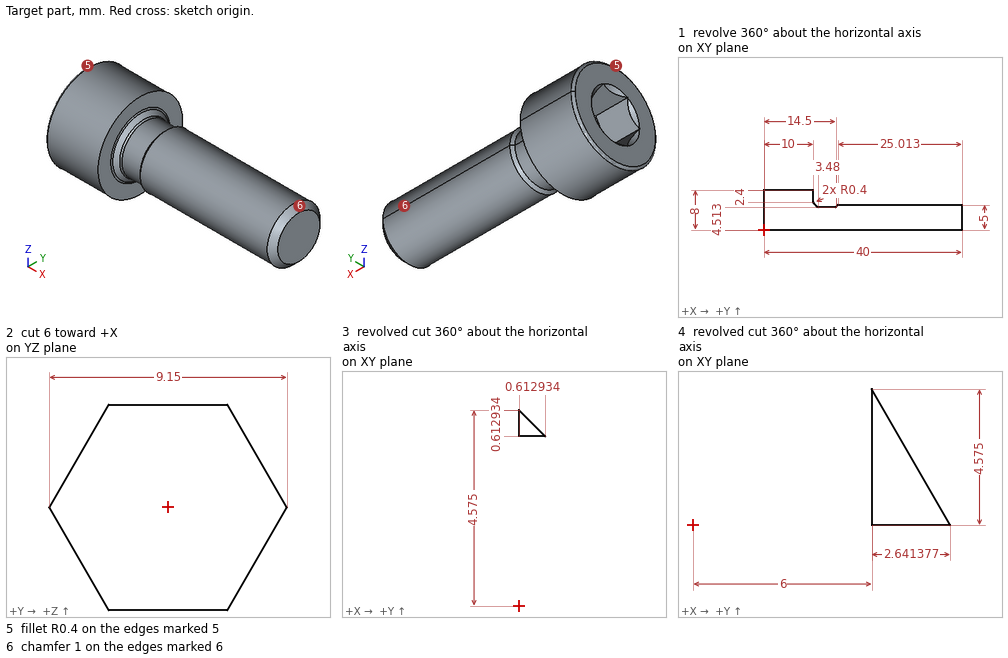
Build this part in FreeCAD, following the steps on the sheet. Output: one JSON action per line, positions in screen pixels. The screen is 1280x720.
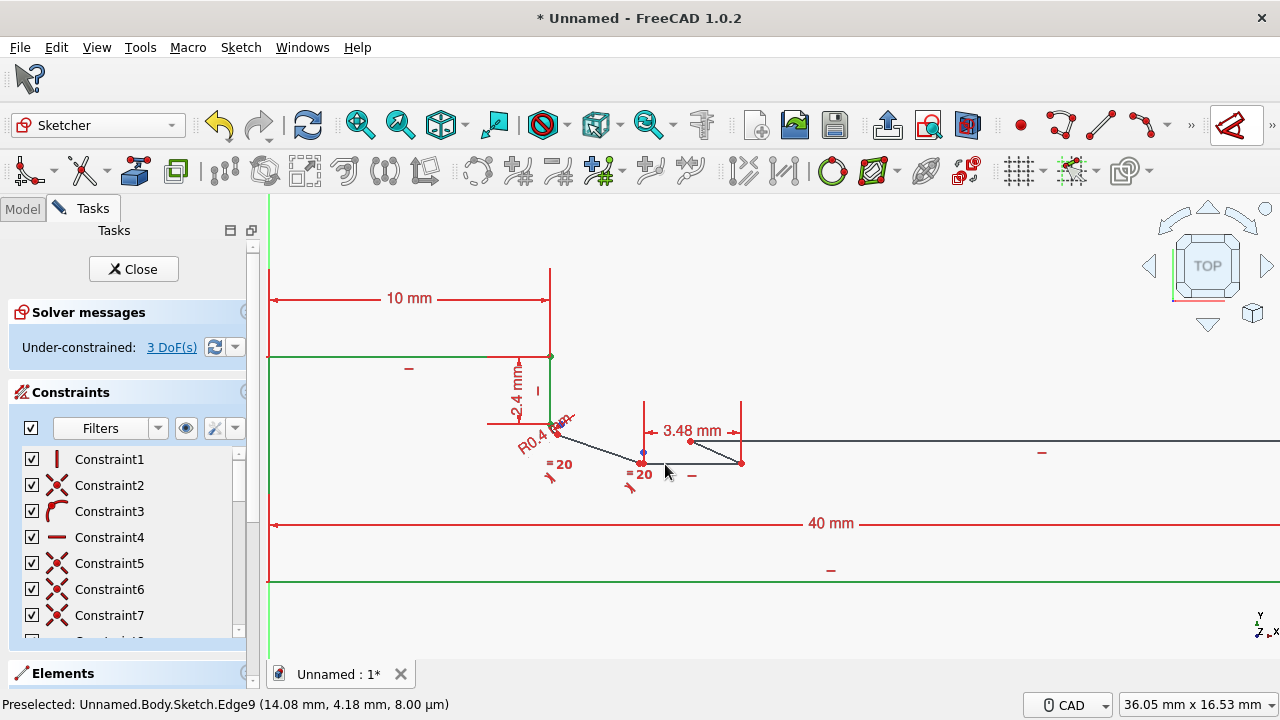
{"action": "left_click", "coordinate": [741, 464]}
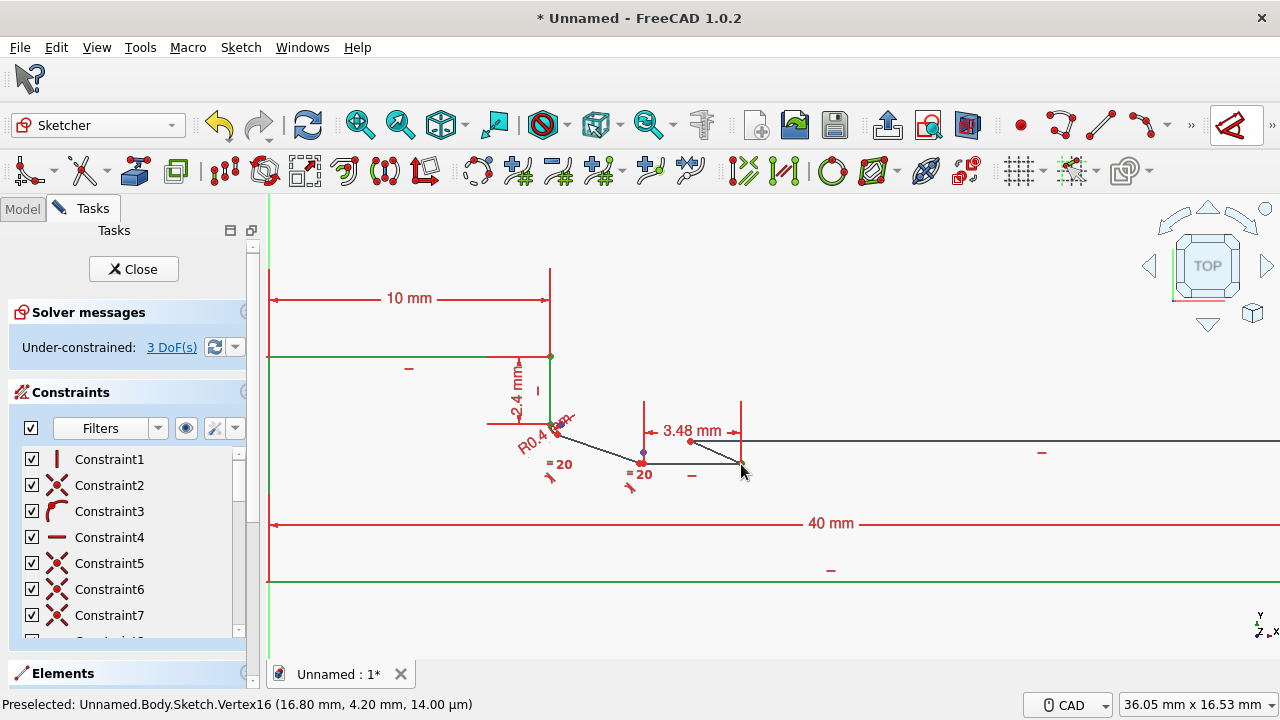
{"action": "key", "text": "l"}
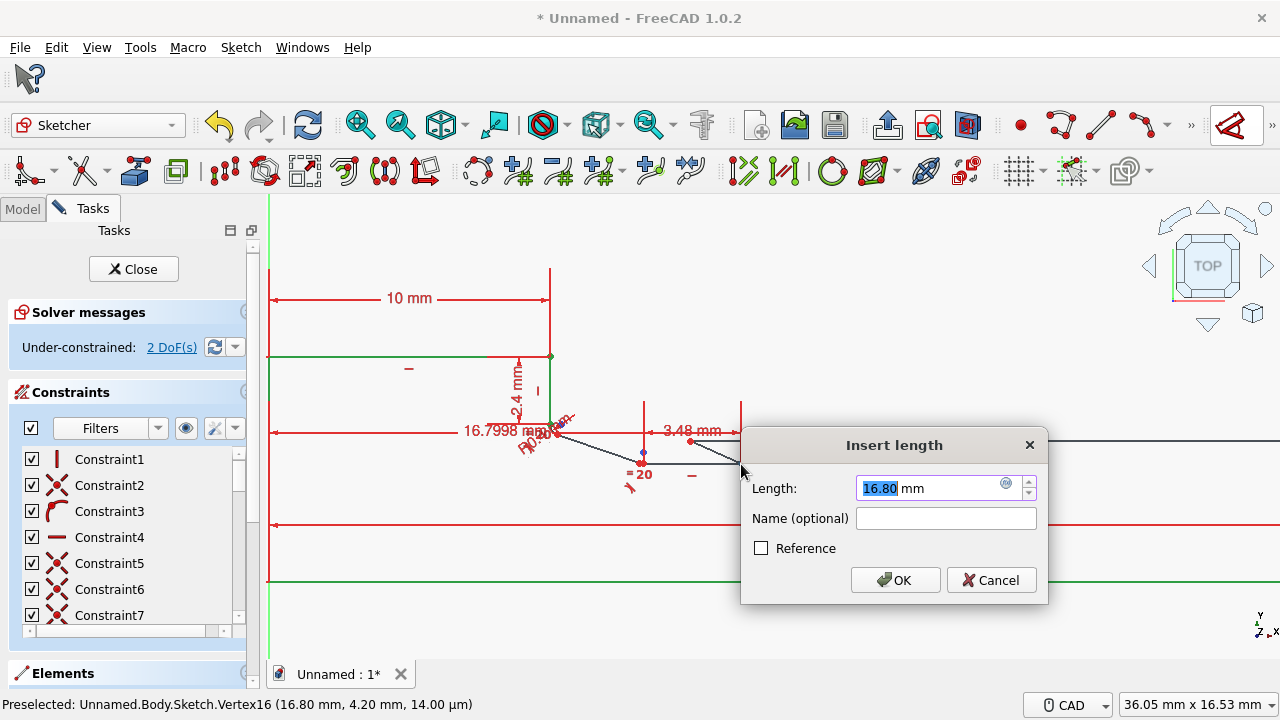
{"action": "type", "text": "14.5"}
{"action": "key", "text": "Return"}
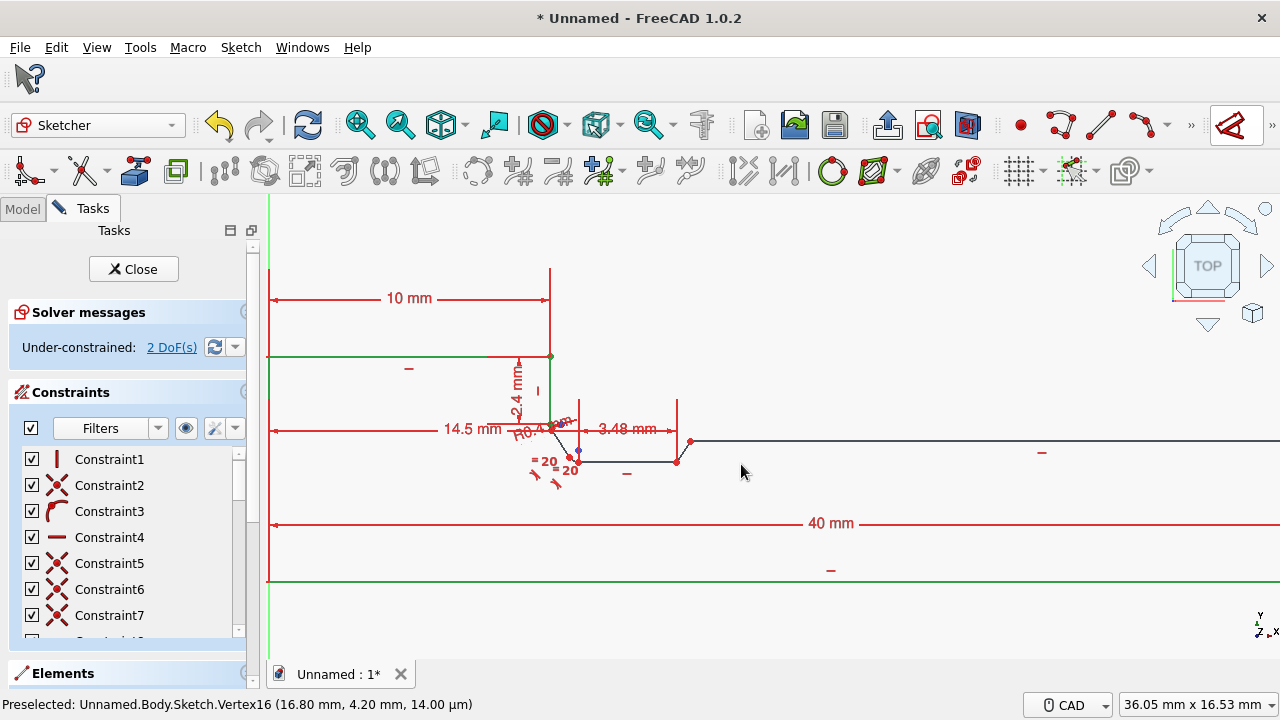
{"action": "left_click", "coordinate": [902, 441]}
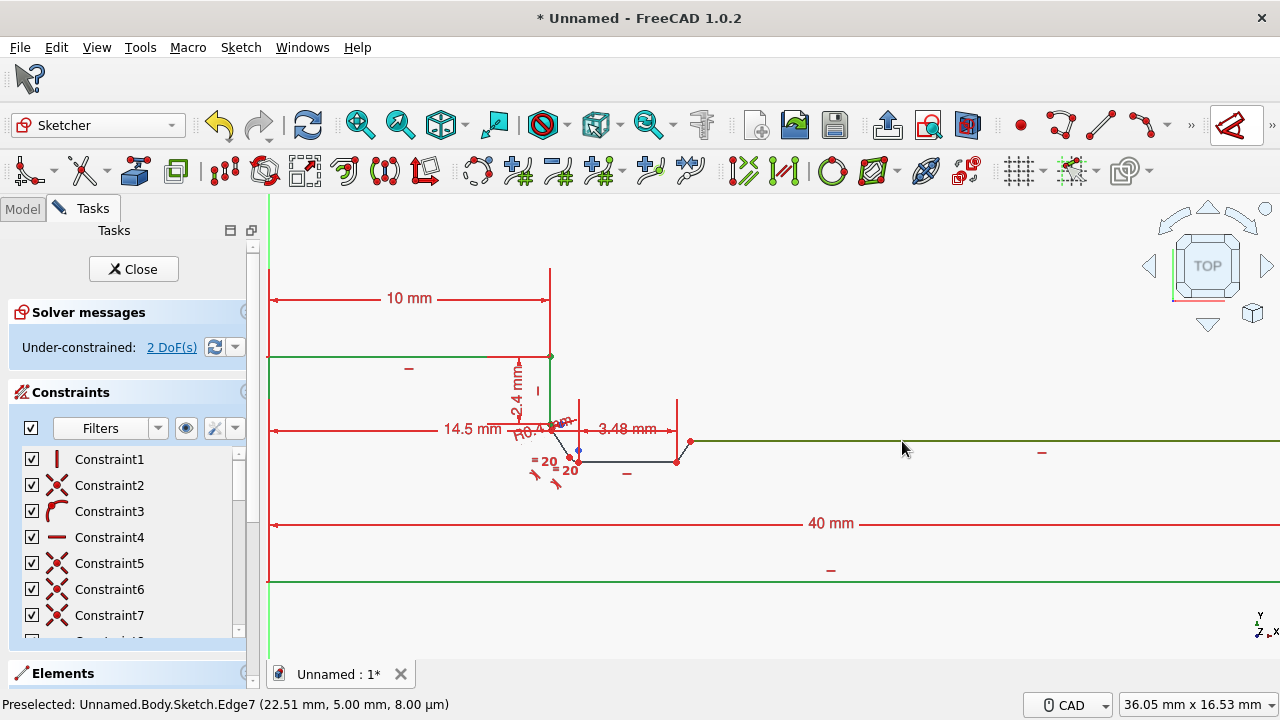
{"action": "left_click", "coordinate": [1258, 126]}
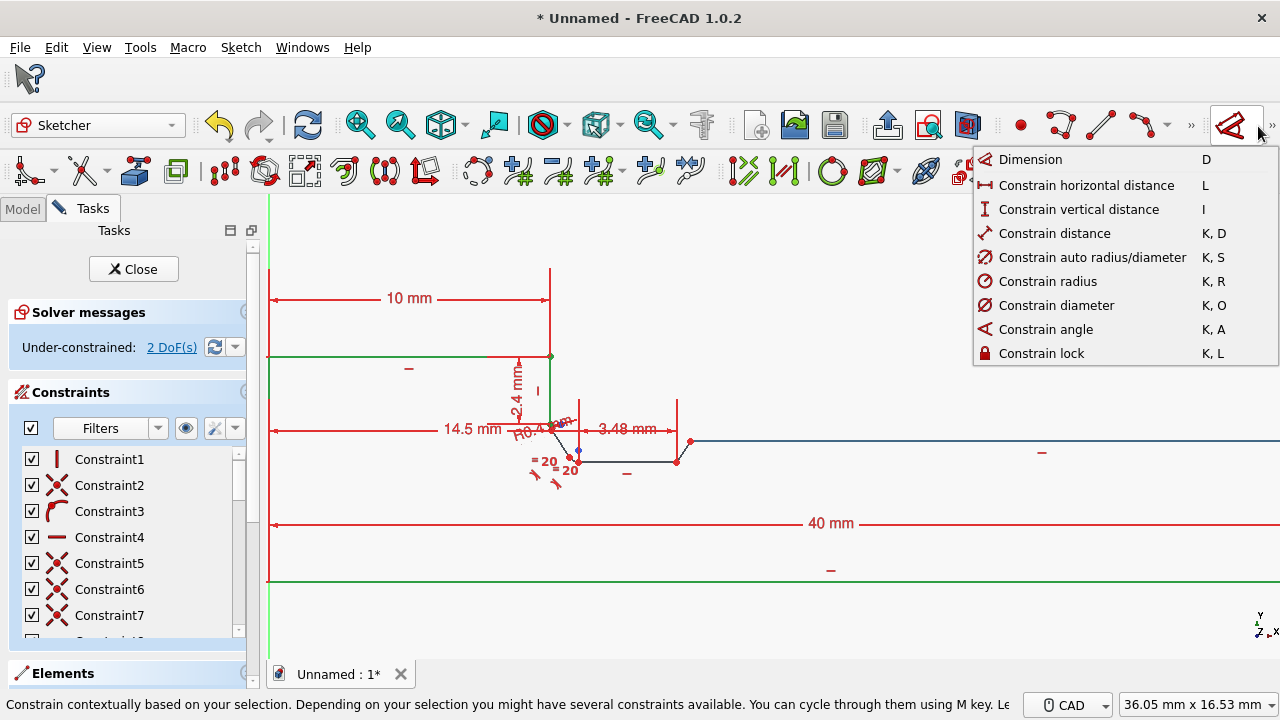
{"action": "left_click", "coordinate": [1126, 185]}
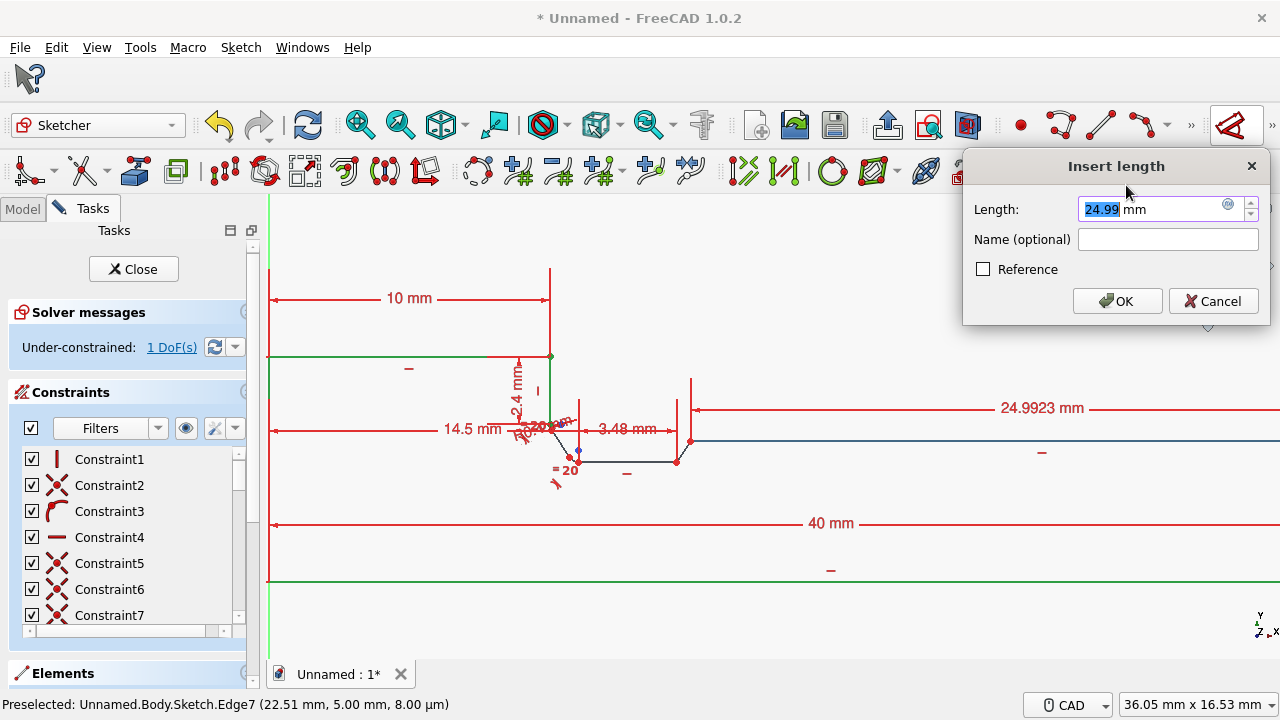
{"action": "type", "text": "25.013"}
{"action": "key", "text": "Return"}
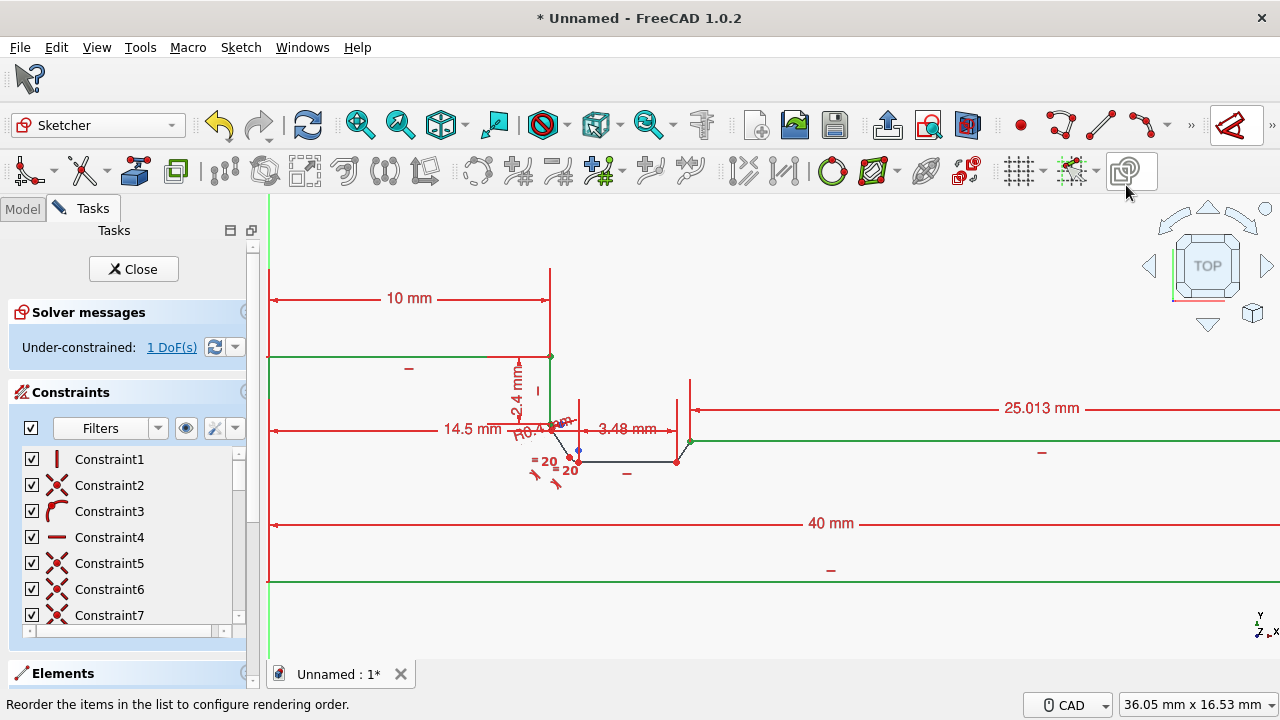
{"action": "left_click", "coordinate": [677, 462]}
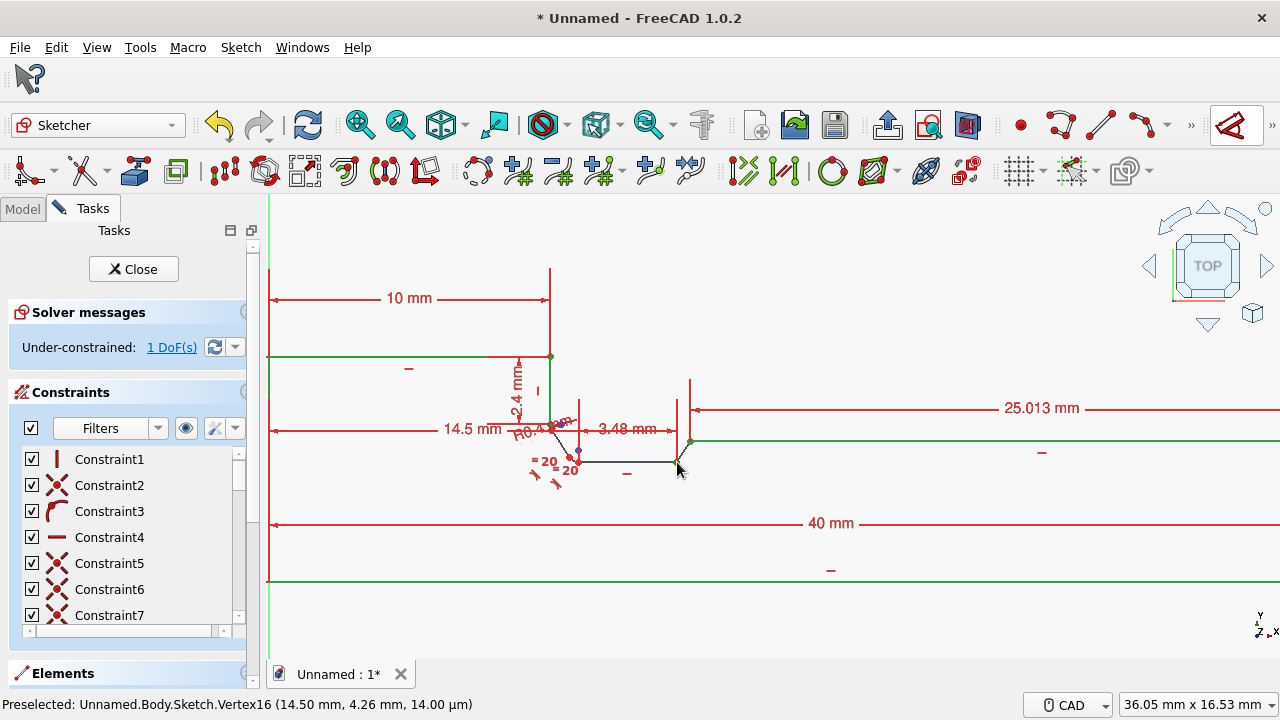
{"action": "key", "text": "i"}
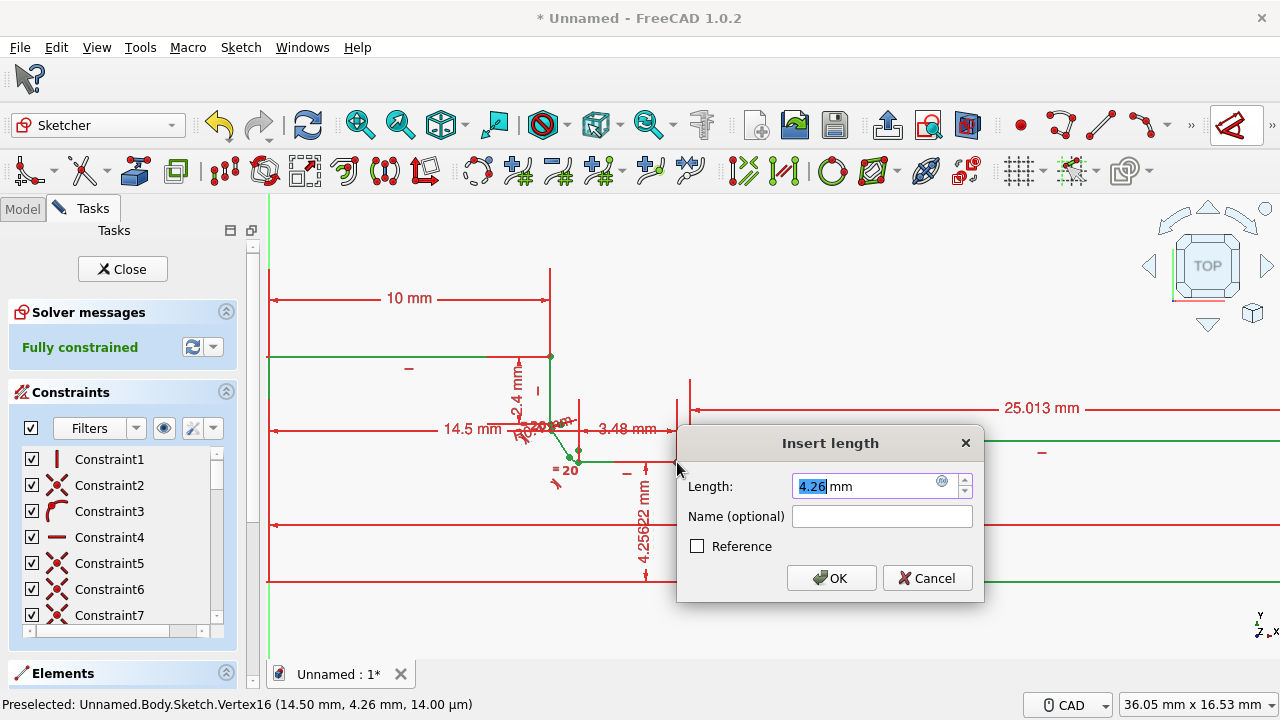
{"action": "type", "text": "4.513"}
{"action": "key", "text": "Return"}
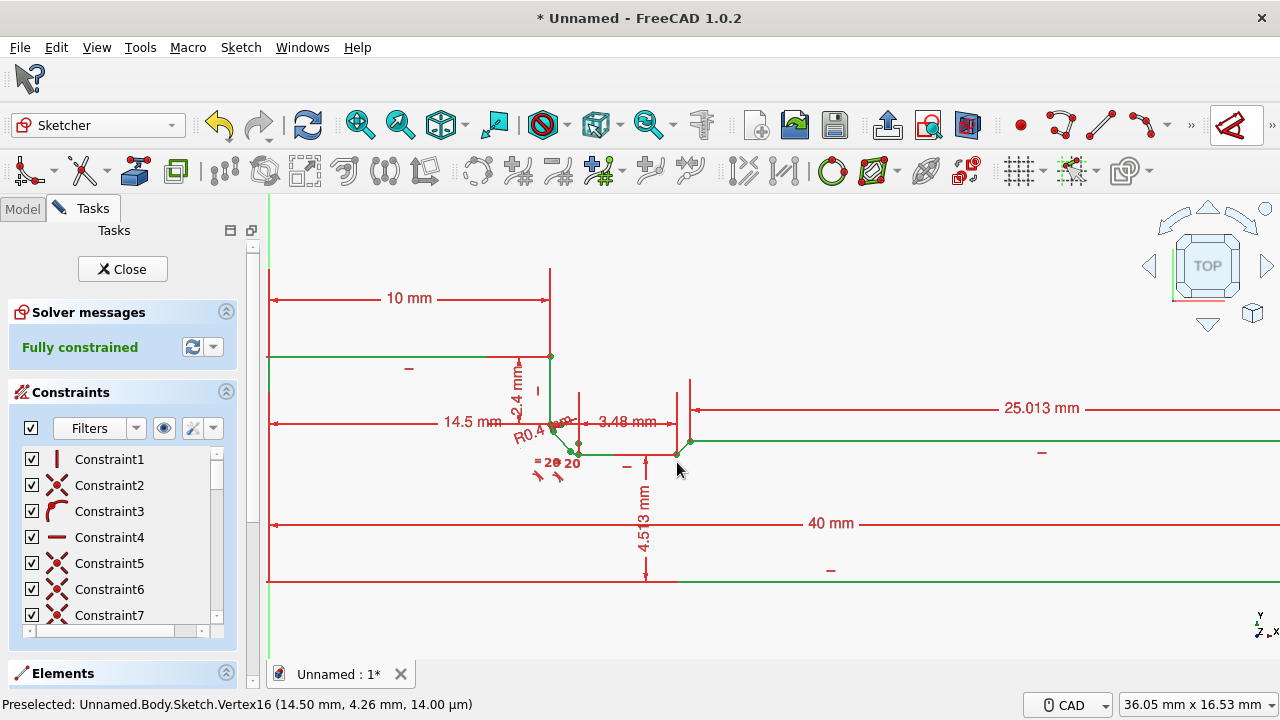
{"action": "left_click", "coordinate": [123, 269]}